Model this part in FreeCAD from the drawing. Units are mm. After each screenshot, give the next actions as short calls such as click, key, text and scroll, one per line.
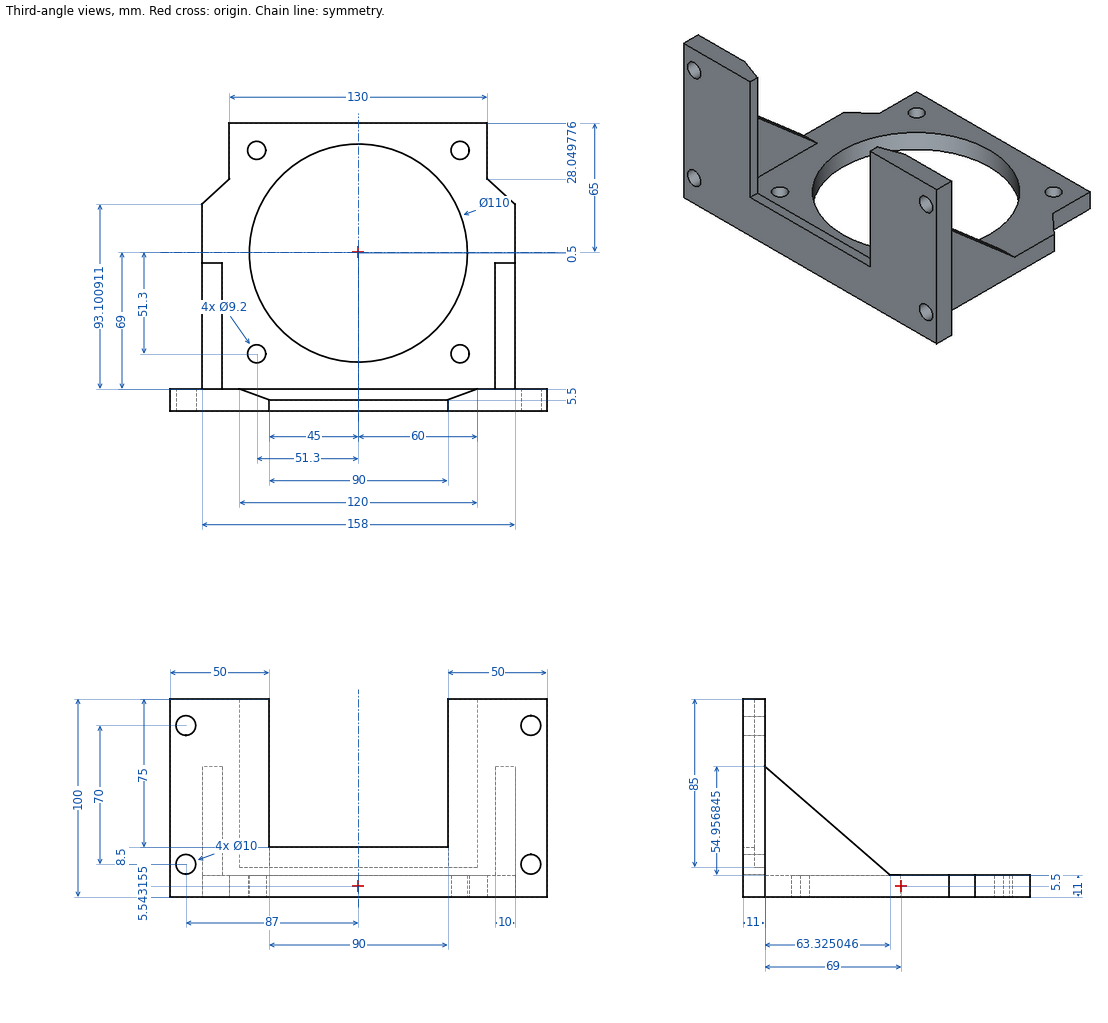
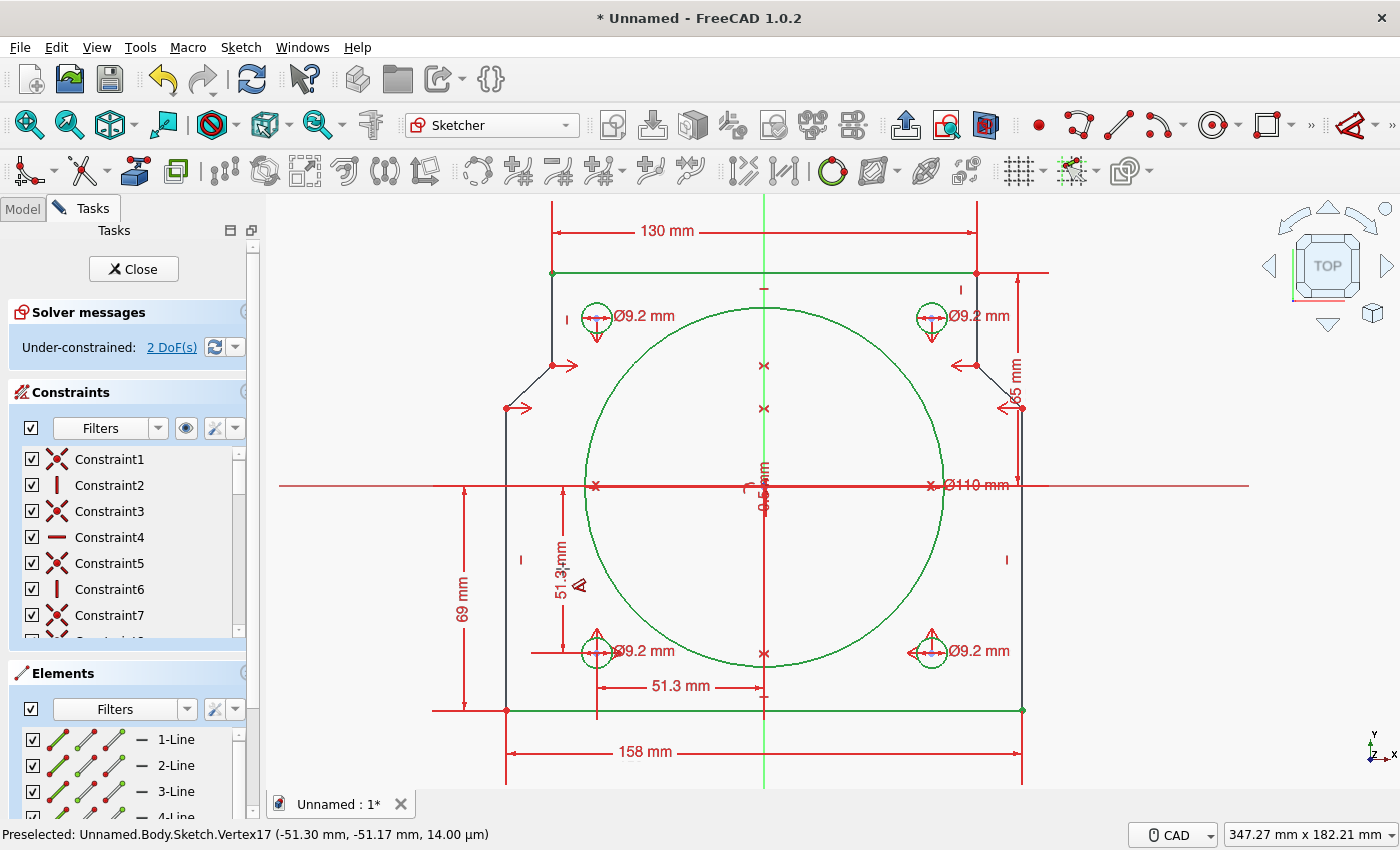
click(506, 499)
click(472, 560)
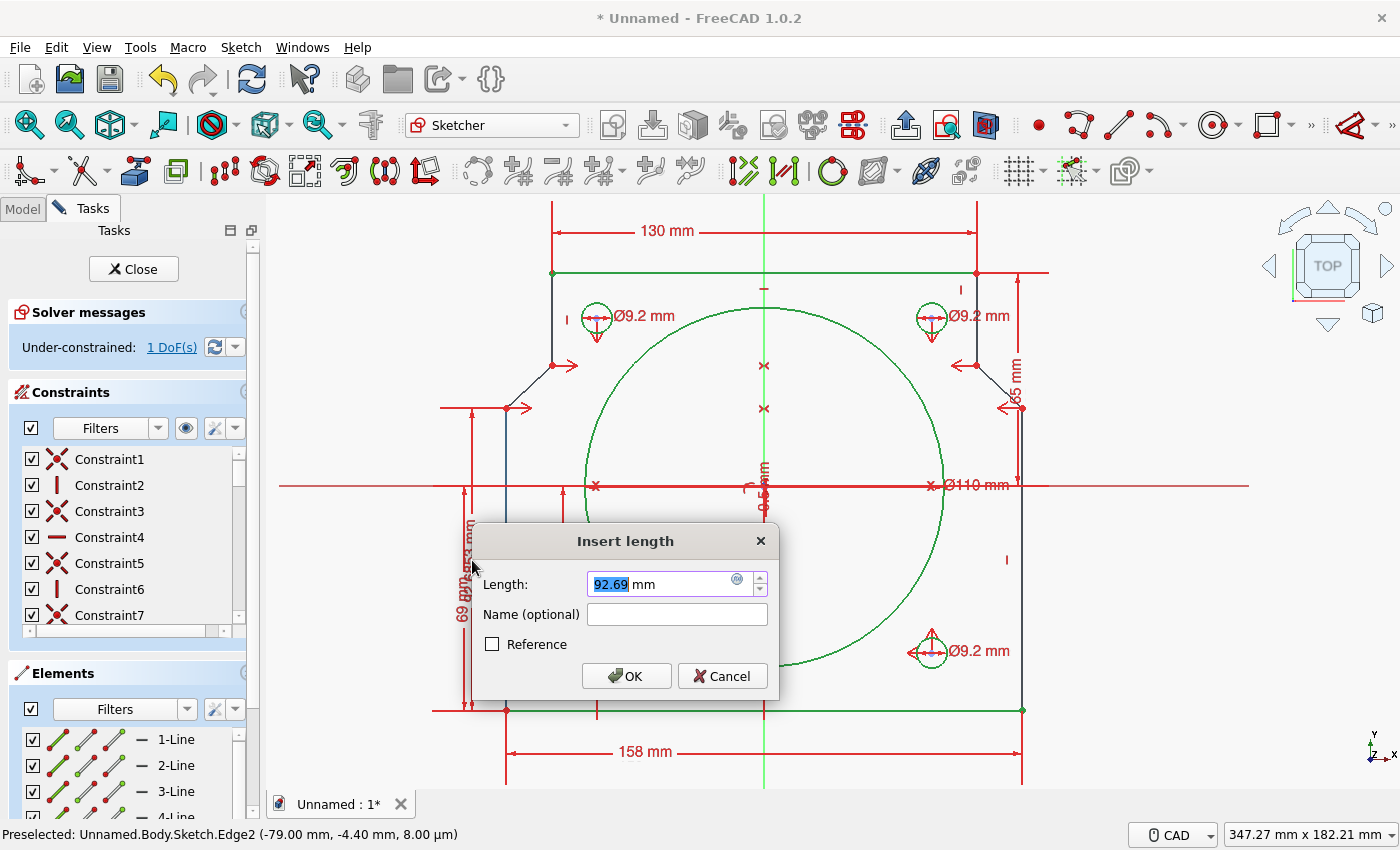
text(93.100911)
key(Return)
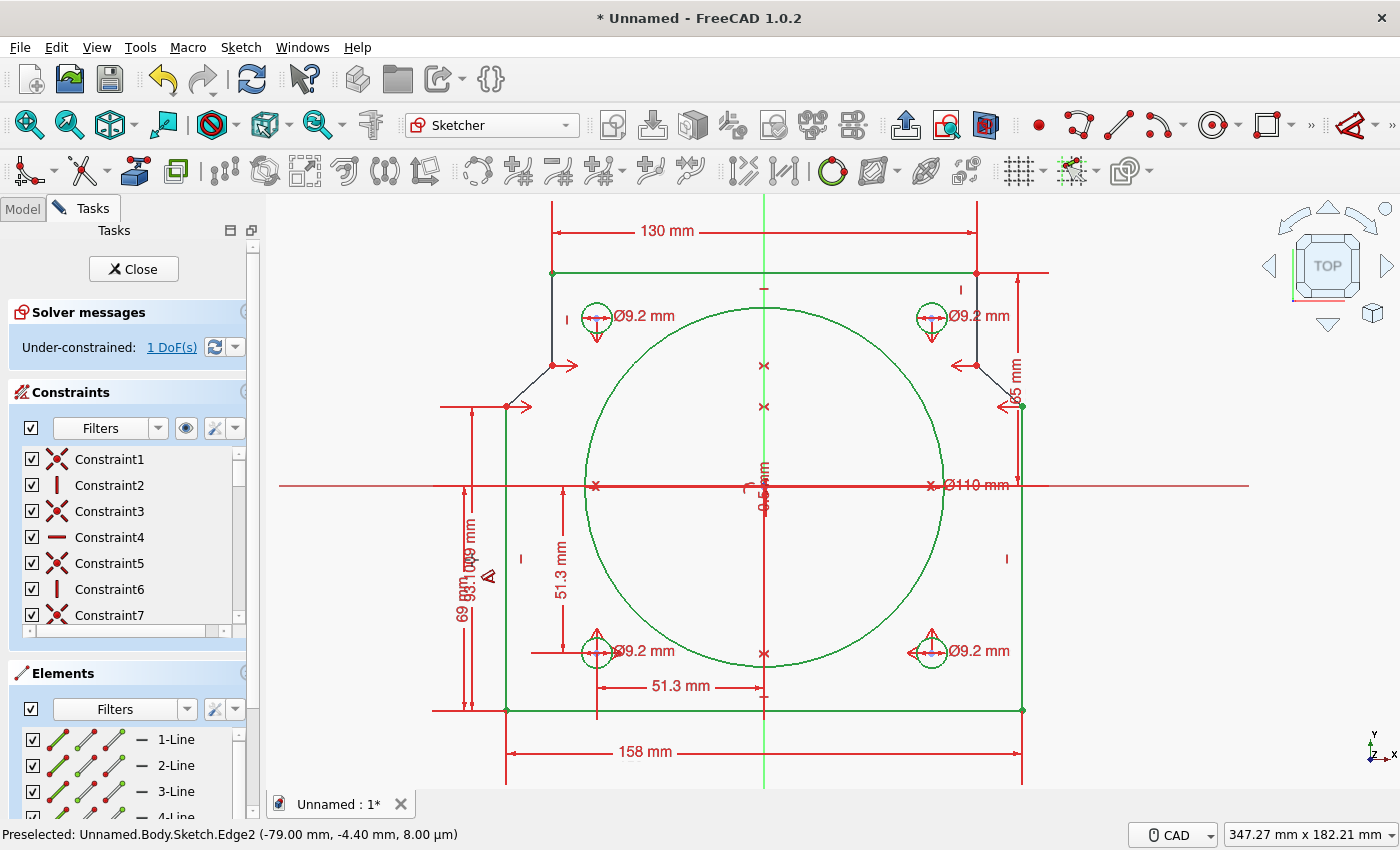
click(977, 338)
click(1011, 320)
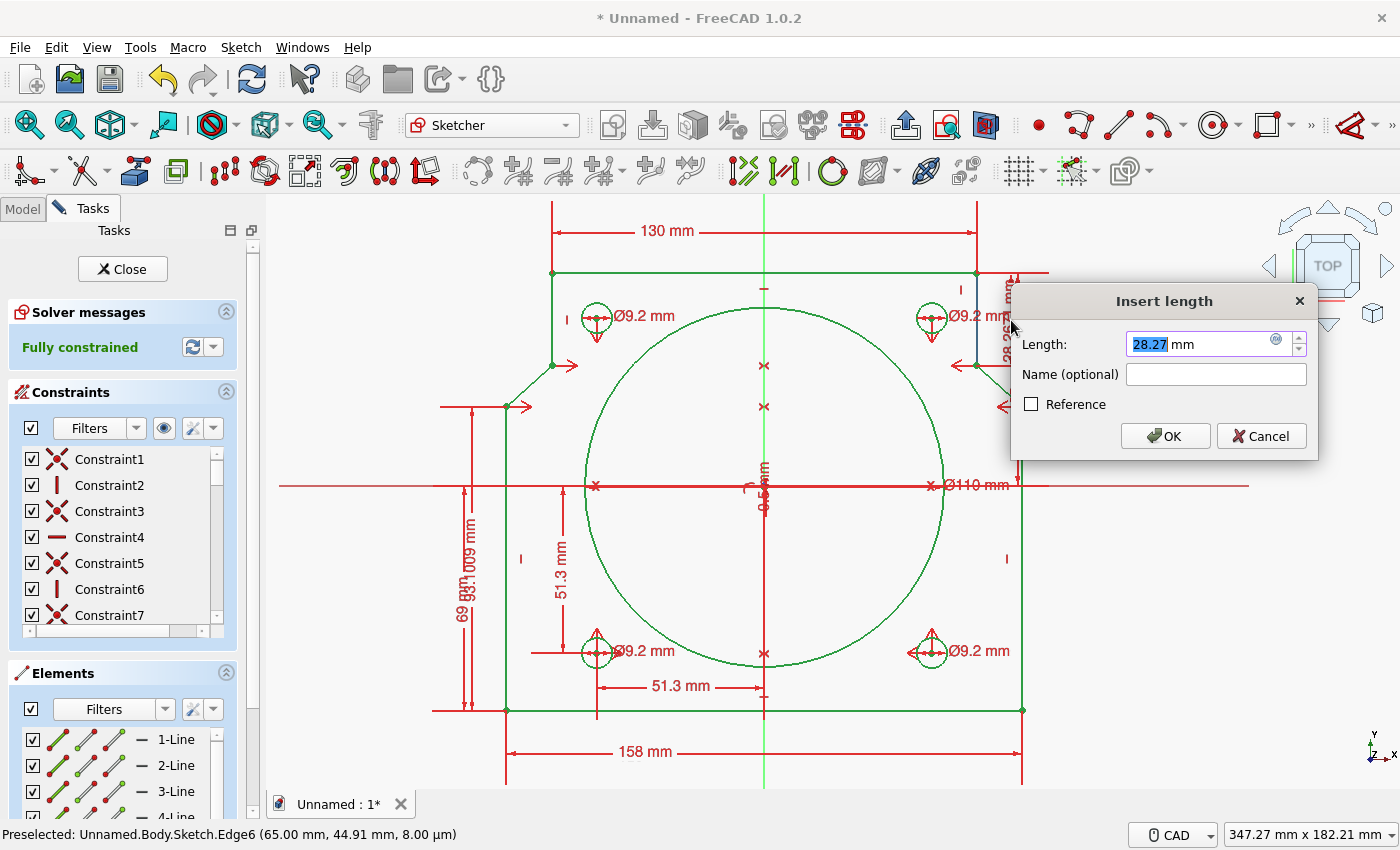
text(28.049776)
key(Return)
key(Escape)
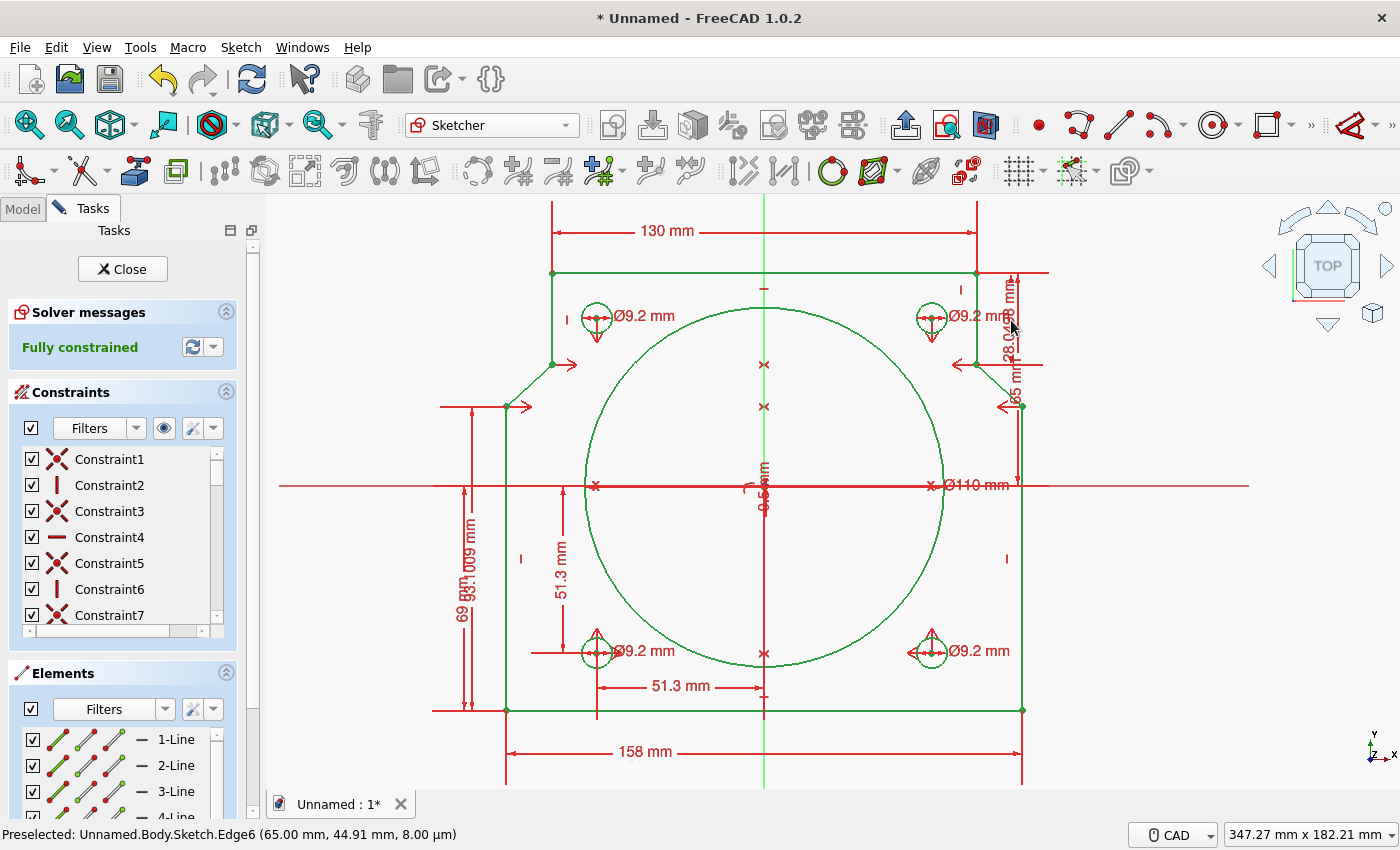
click(123, 269)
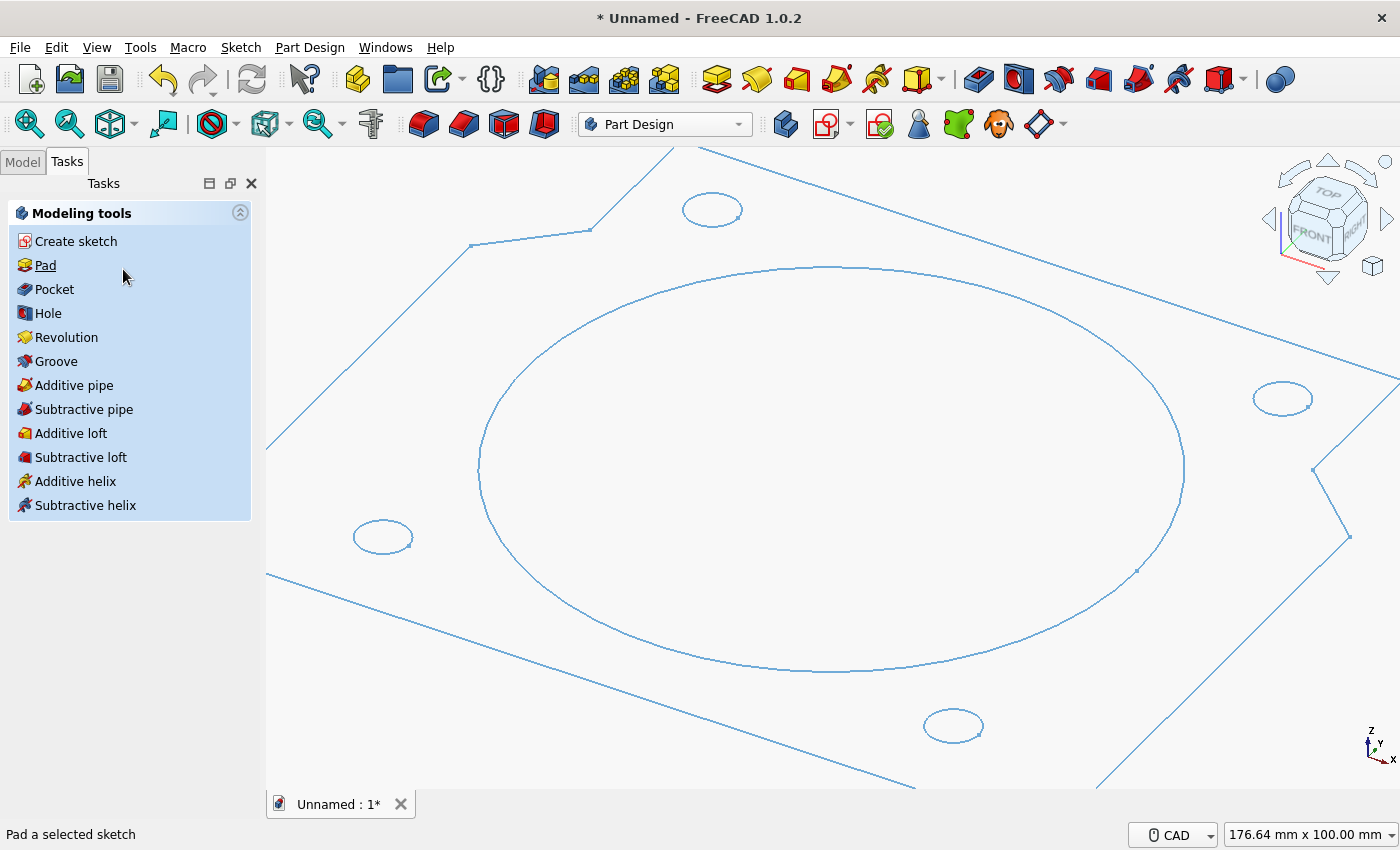
click(718, 80)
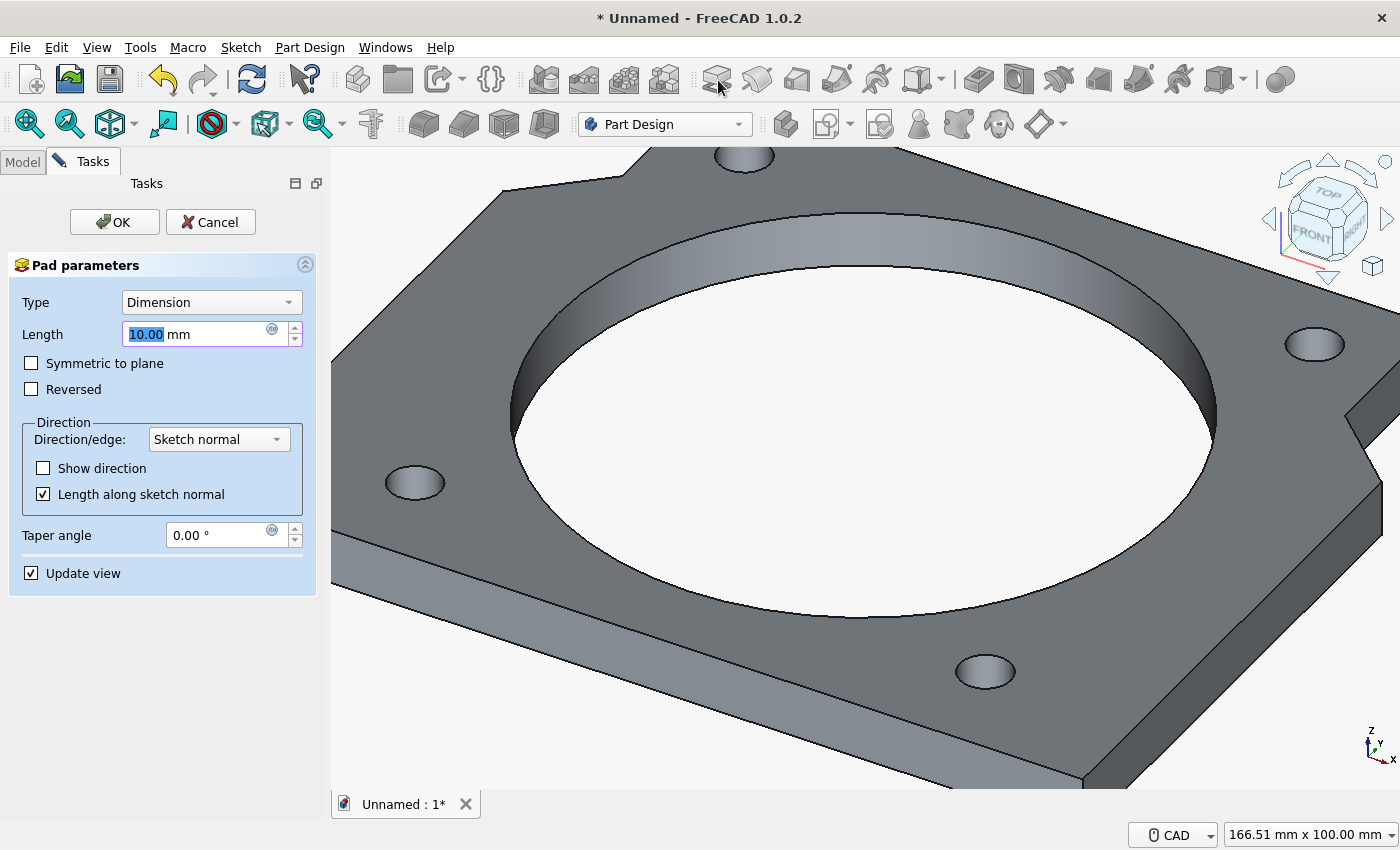
text(11)
key(Tab)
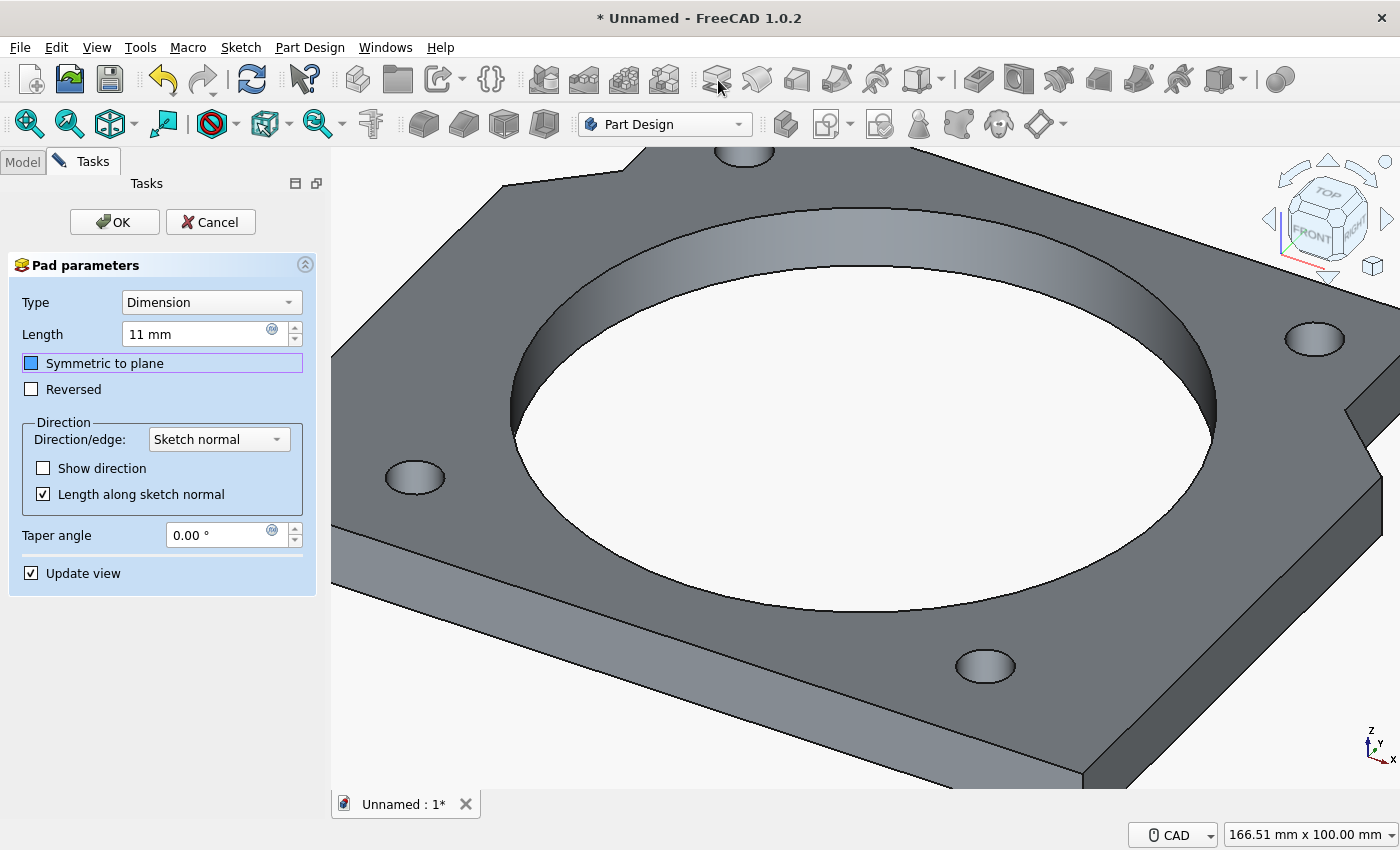
click(30, 363)